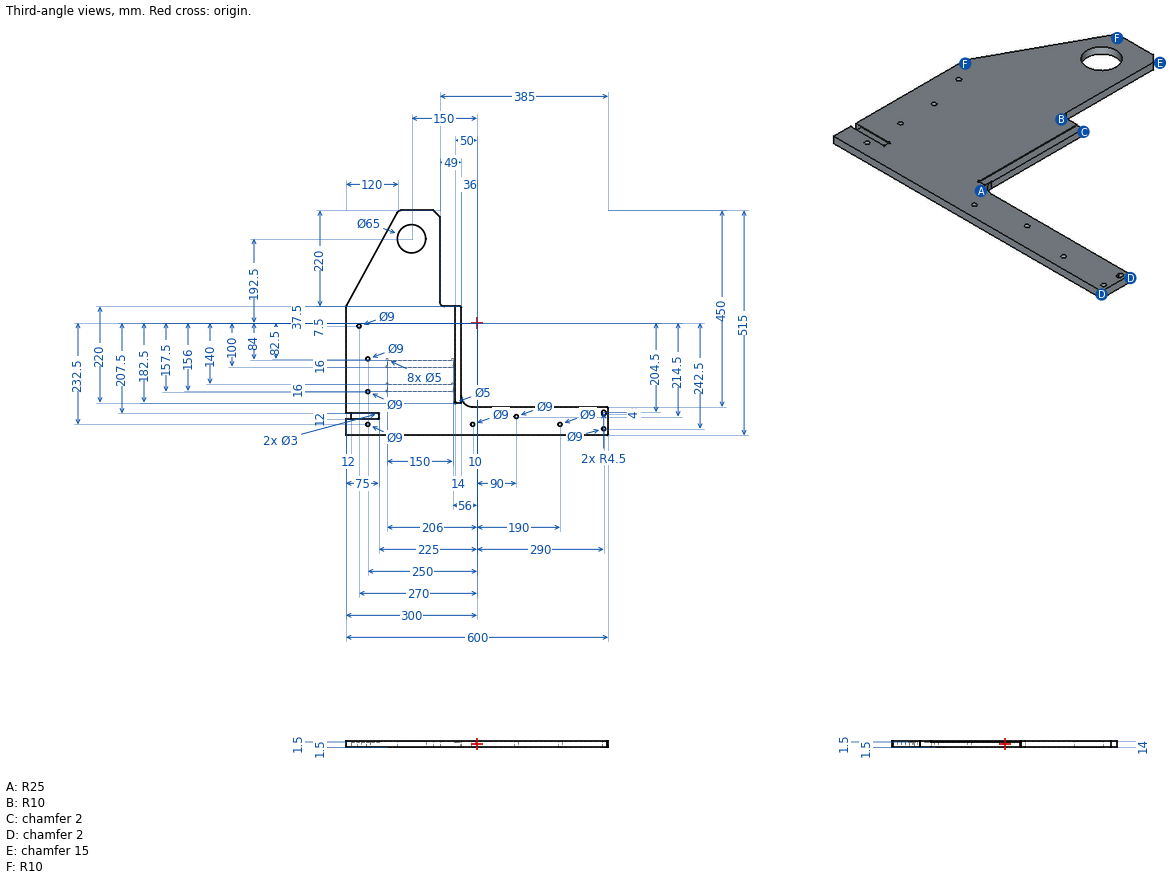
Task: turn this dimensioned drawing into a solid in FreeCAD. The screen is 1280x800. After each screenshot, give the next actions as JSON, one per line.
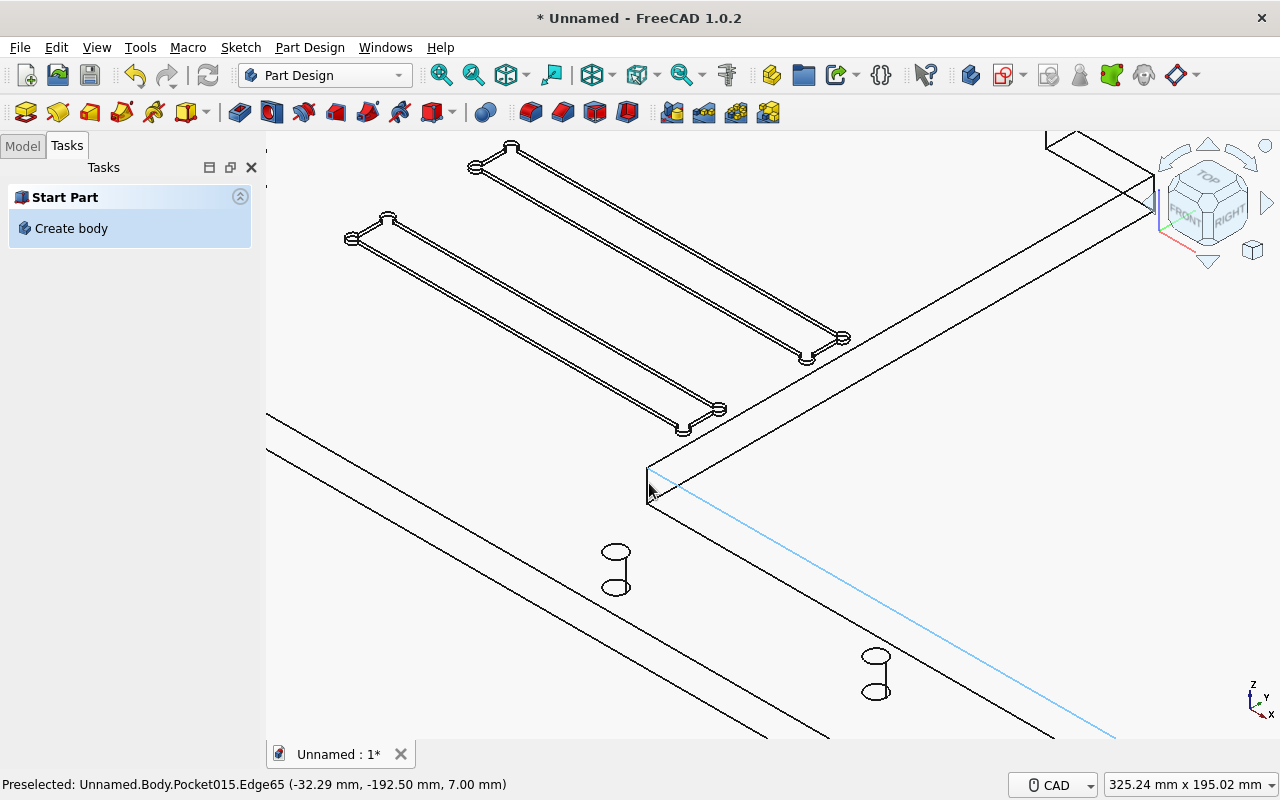
{"action": "left_click", "coordinate": [647, 485]}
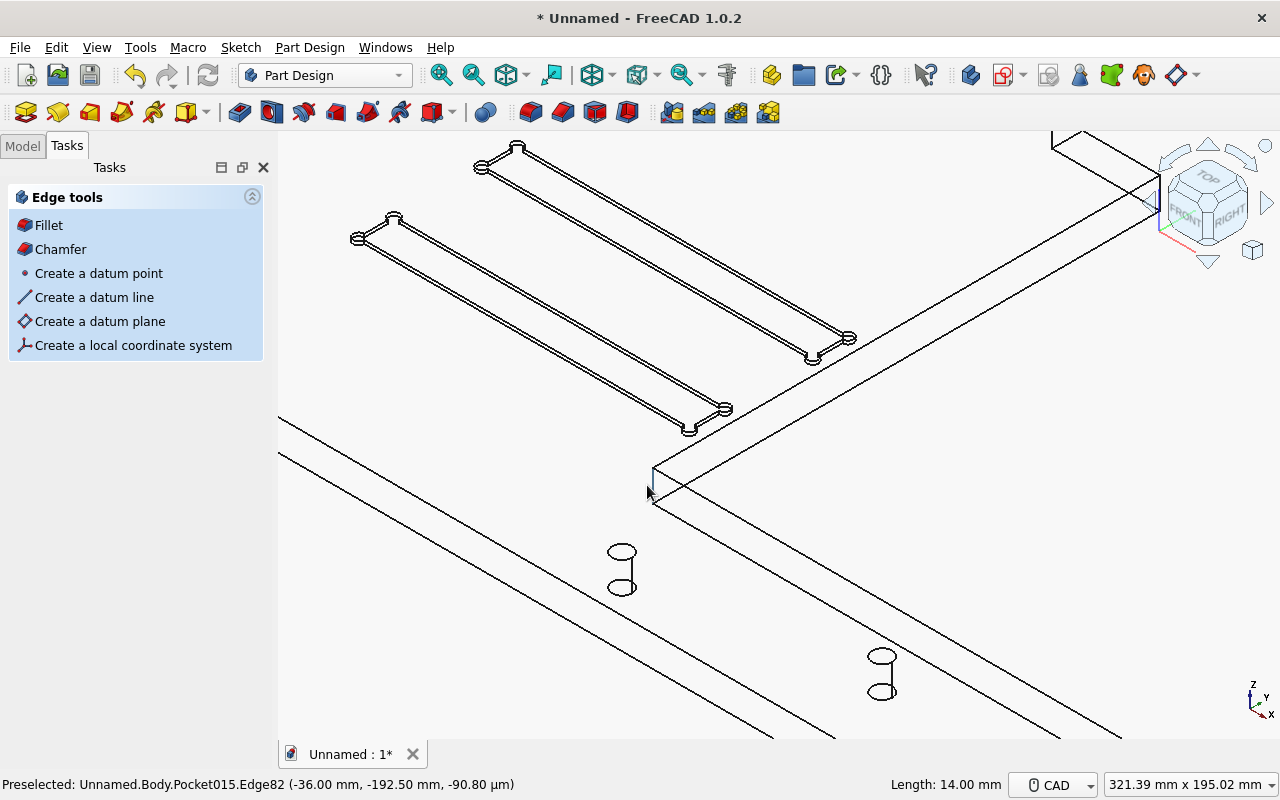
{"action": "key", "text": "v 1"}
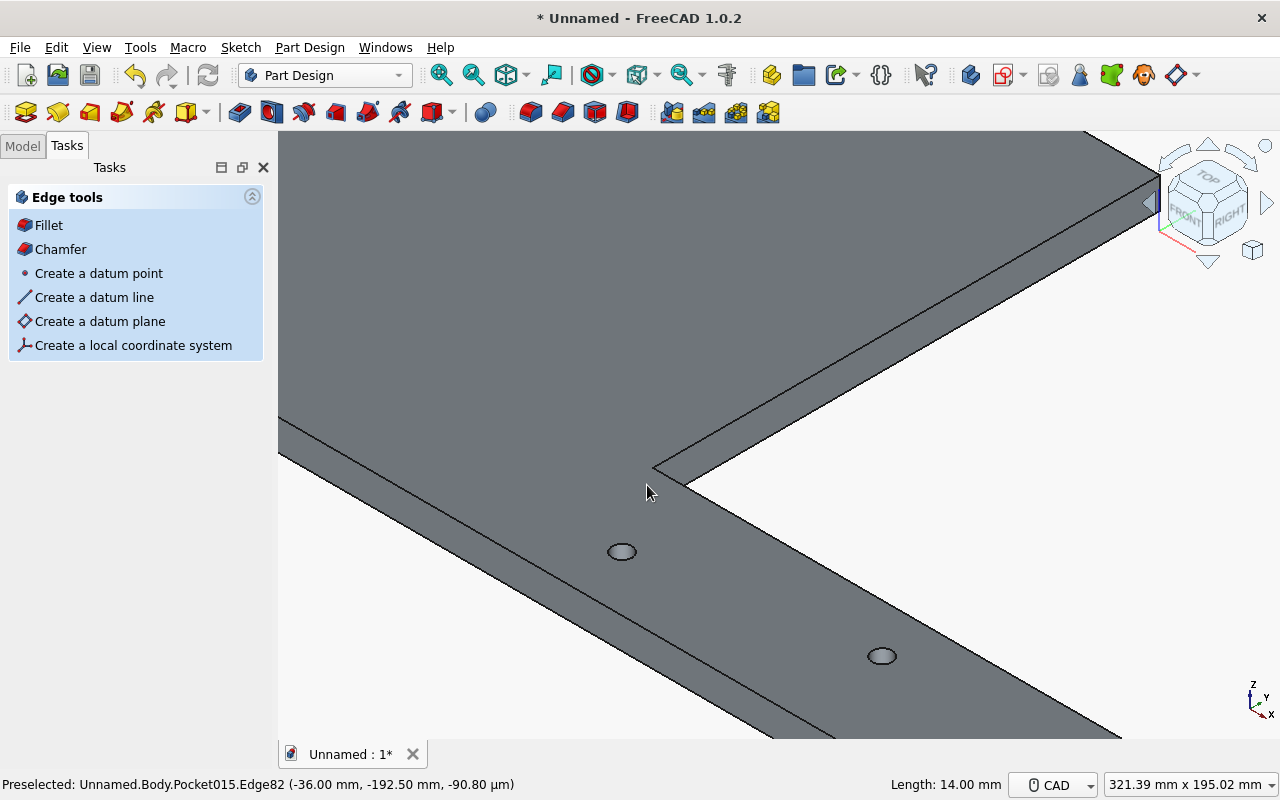
{"action": "left_click", "coordinate": [532, 112]}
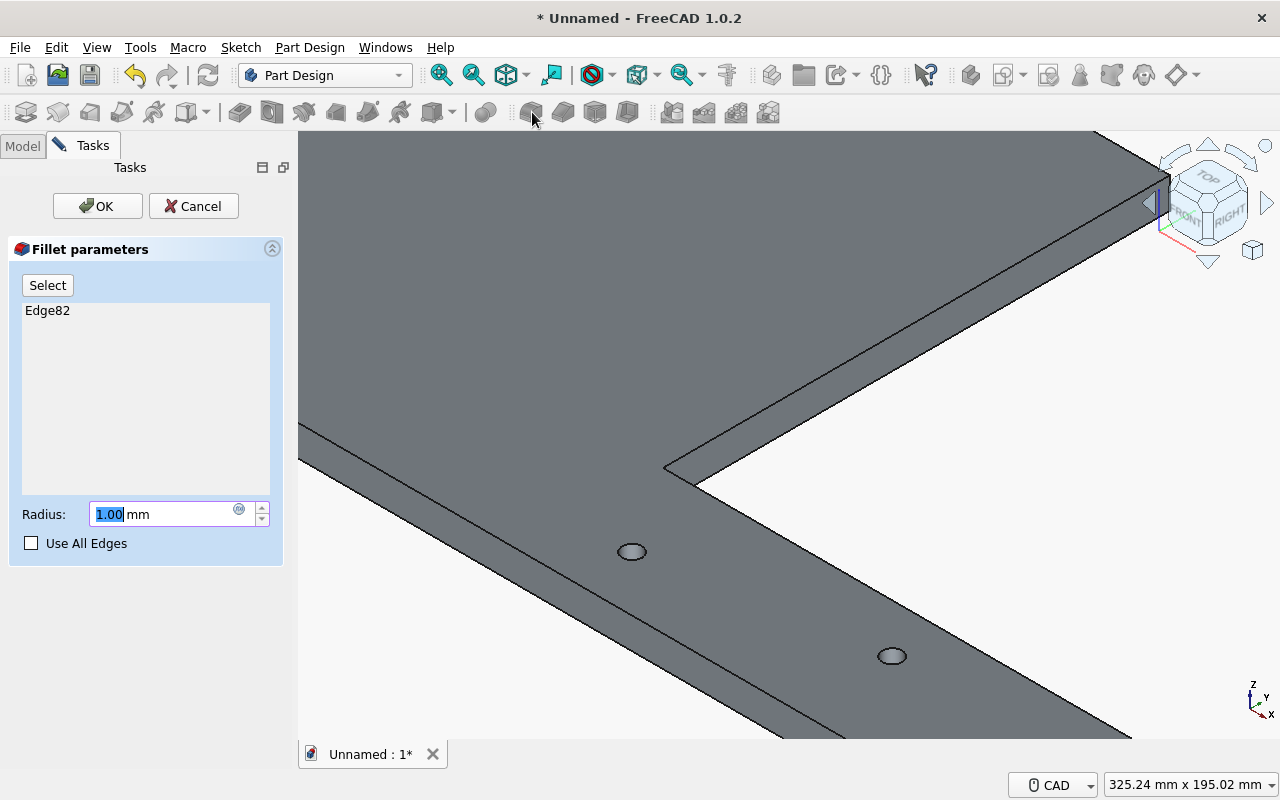
{"action": "type", "text": "25"}
{"action": "key", "text": "Tab"}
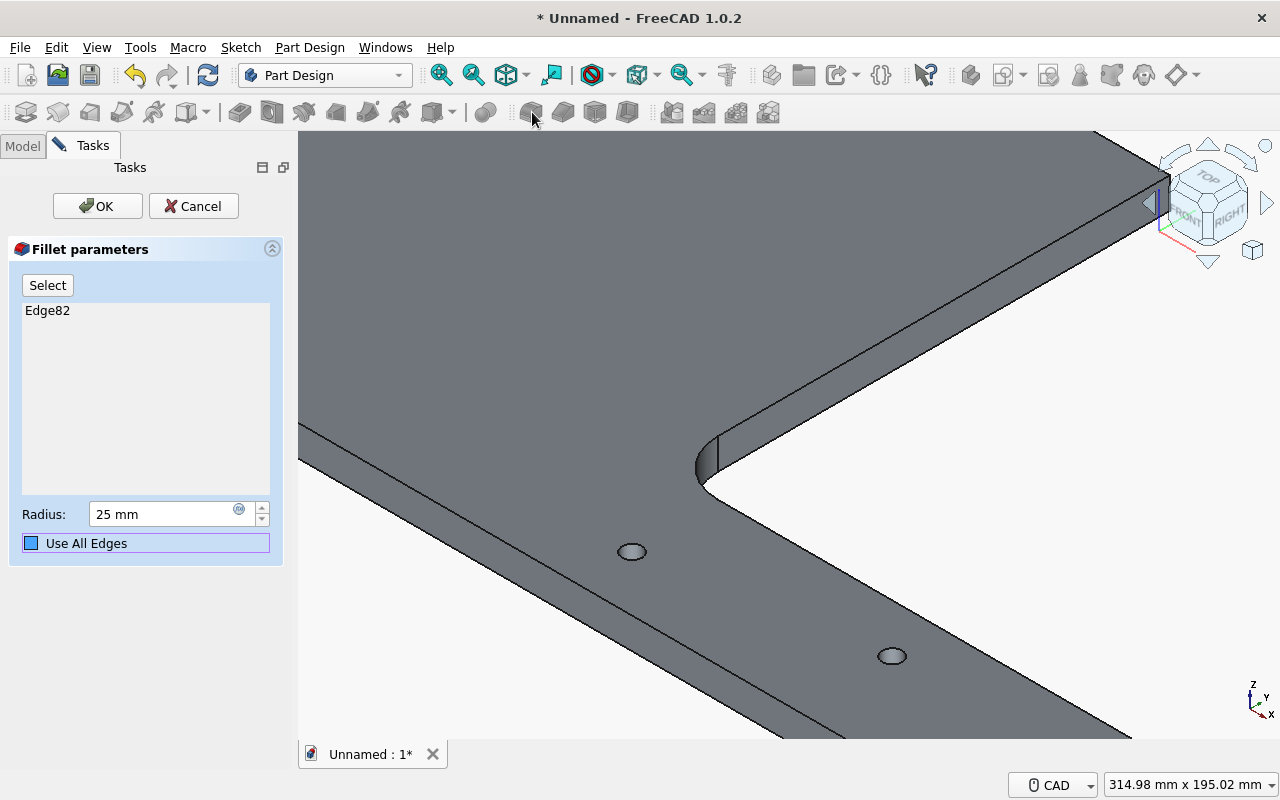
{"action": "left_click", "coordinate": [98, 206]}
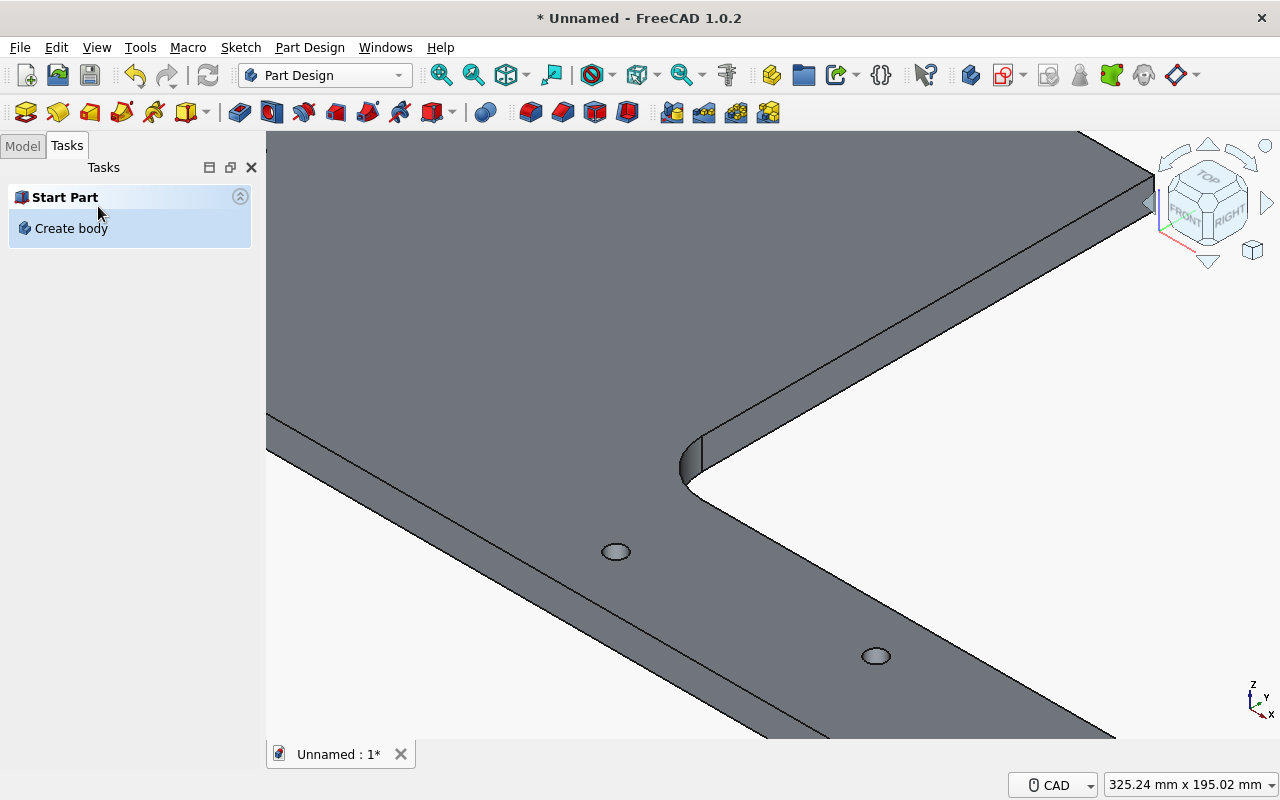
{"action": "left_click", "coordinate": [442, 76]}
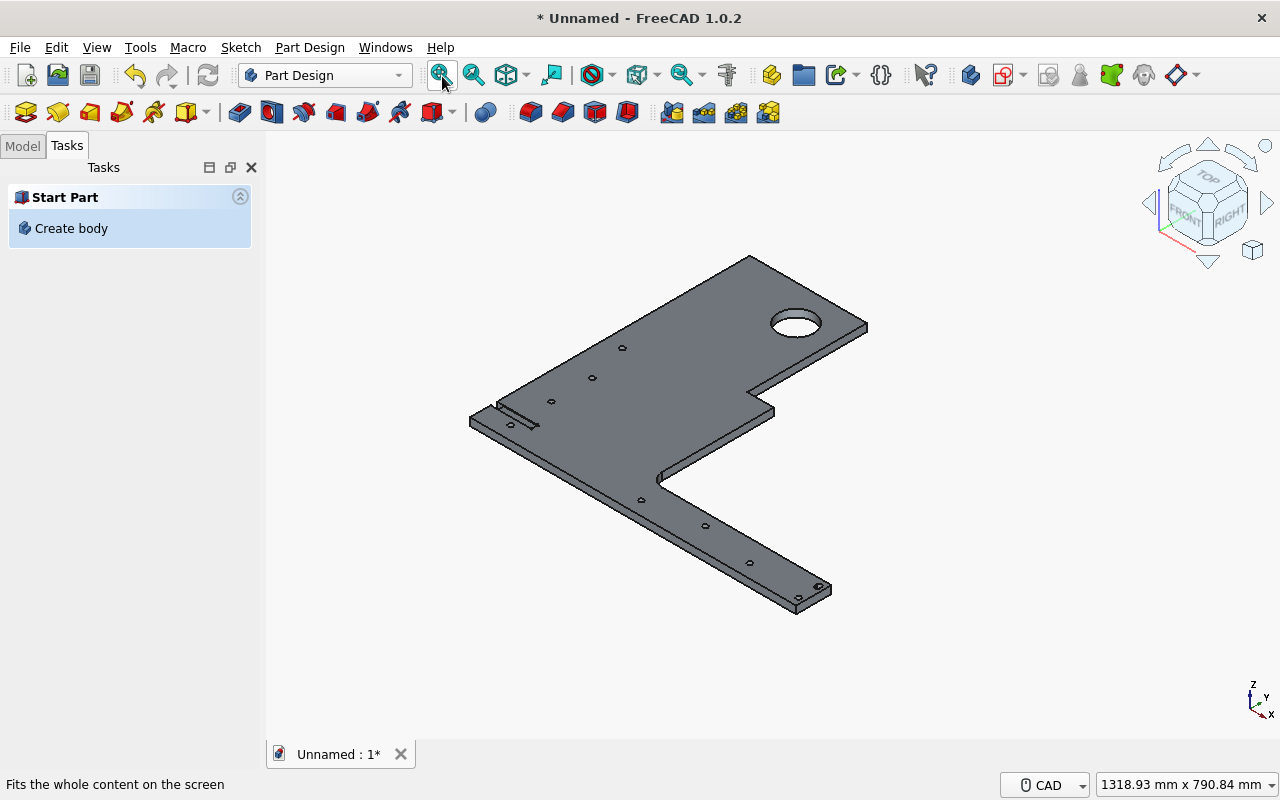
{"action": "left_click", "coordinate": [680, 376]}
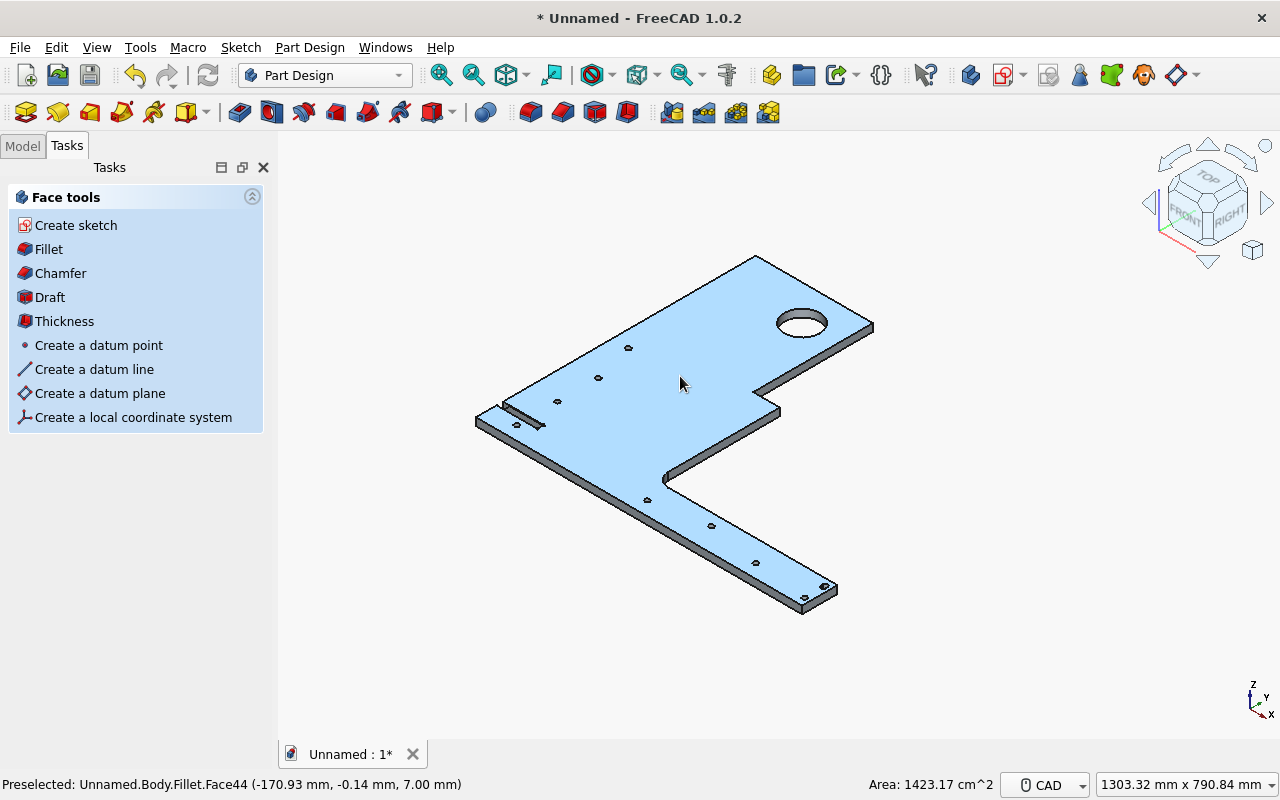
{"action": "left_click", "coordinate": [1004, 76]}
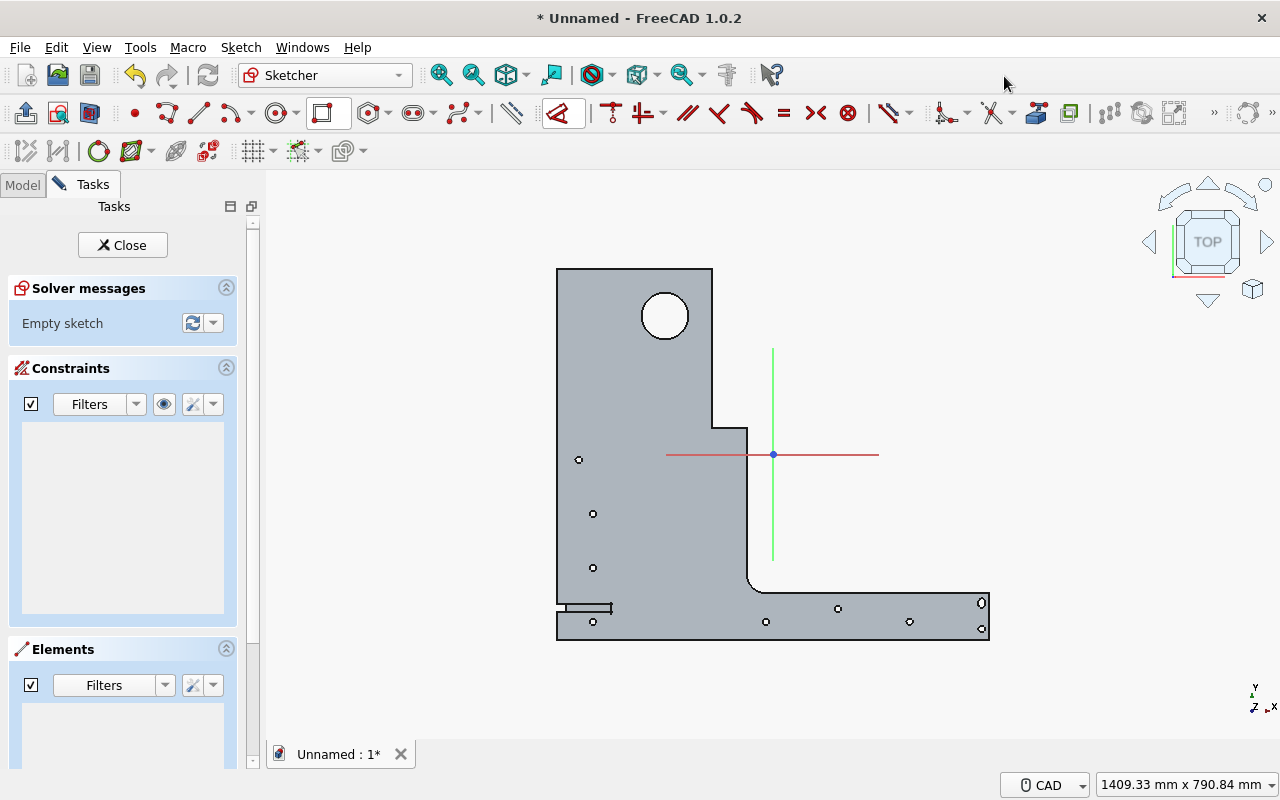
{"action": "scroll", "coordinate": [796, 549], "scroll_direction": "up", "scroll_amount": 4}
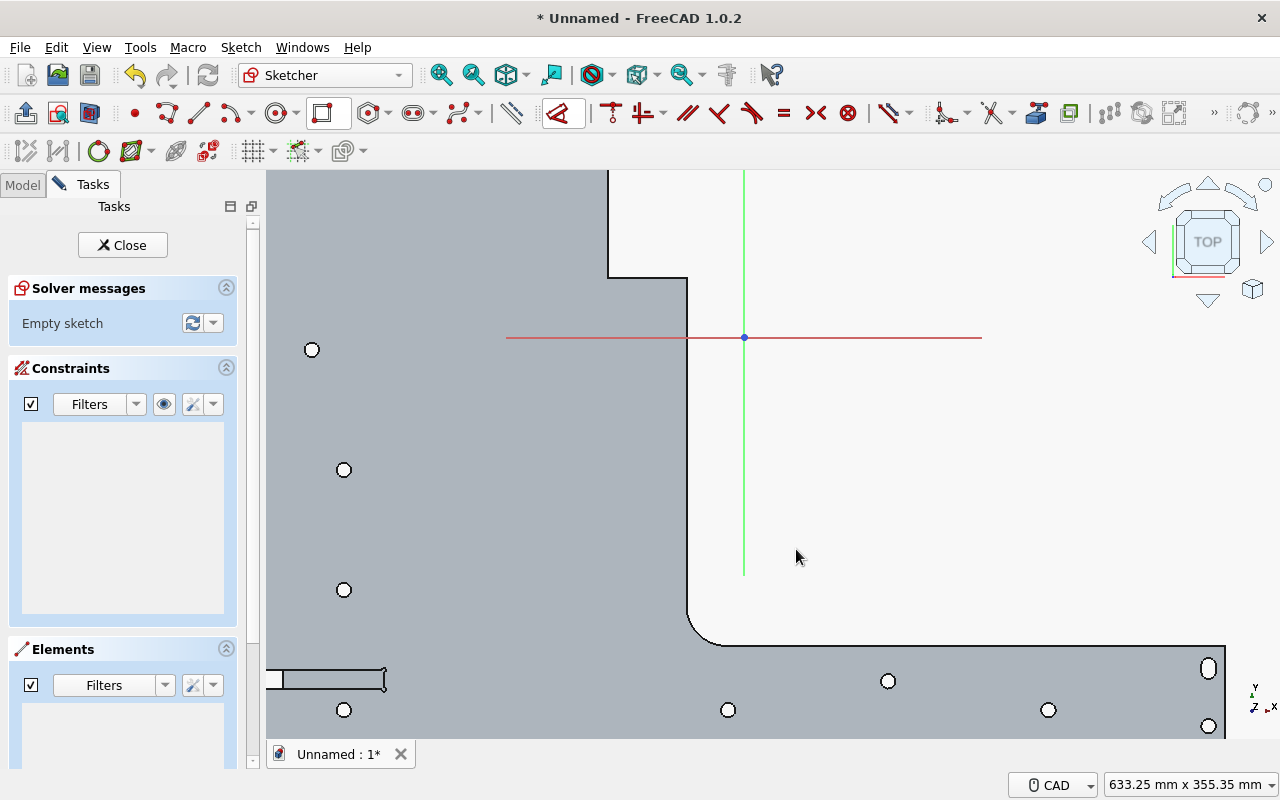
{"action": "left_click", "coordinate": [322, 114]}